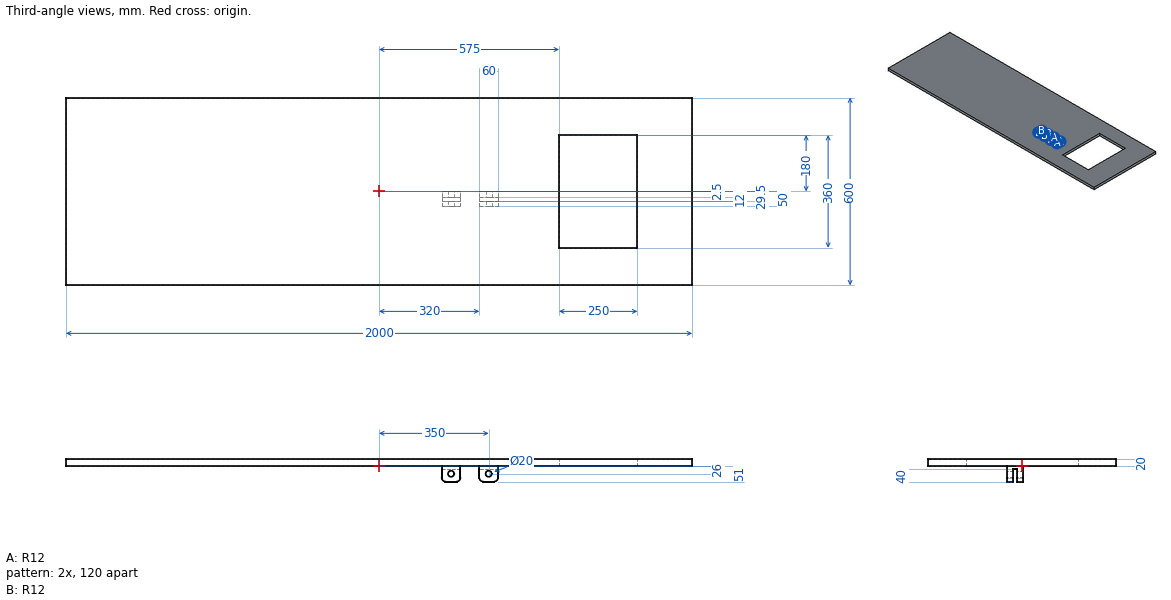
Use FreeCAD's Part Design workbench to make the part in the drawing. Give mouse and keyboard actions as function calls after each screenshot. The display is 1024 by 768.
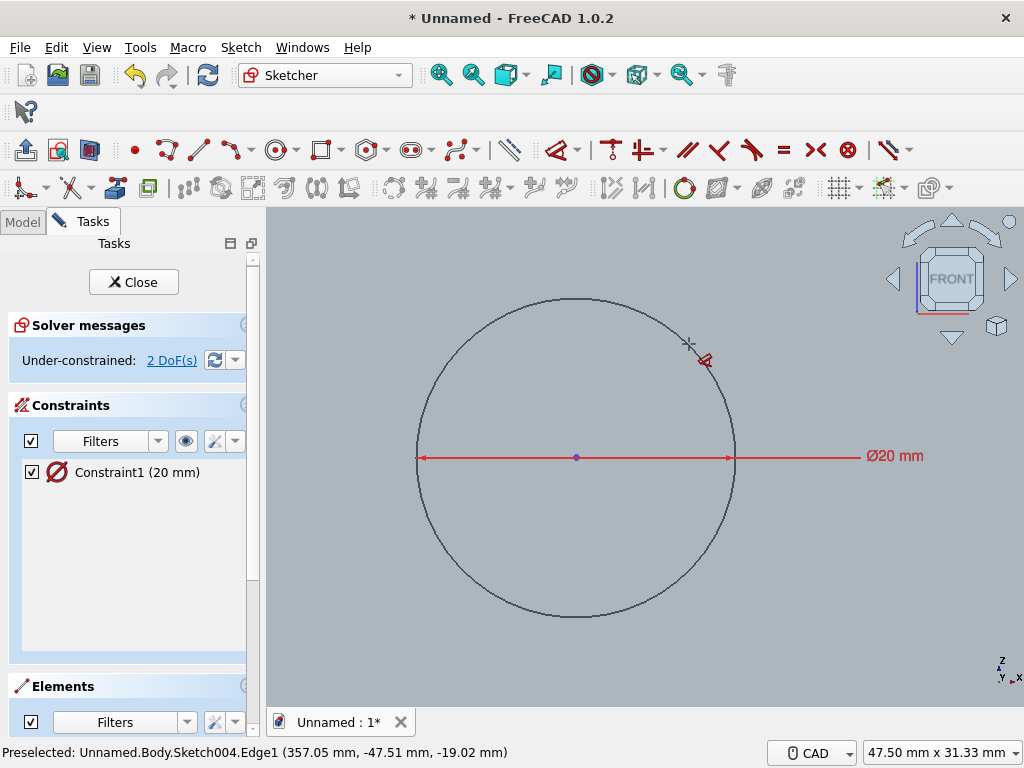
click(576, 458)
click(610, 347)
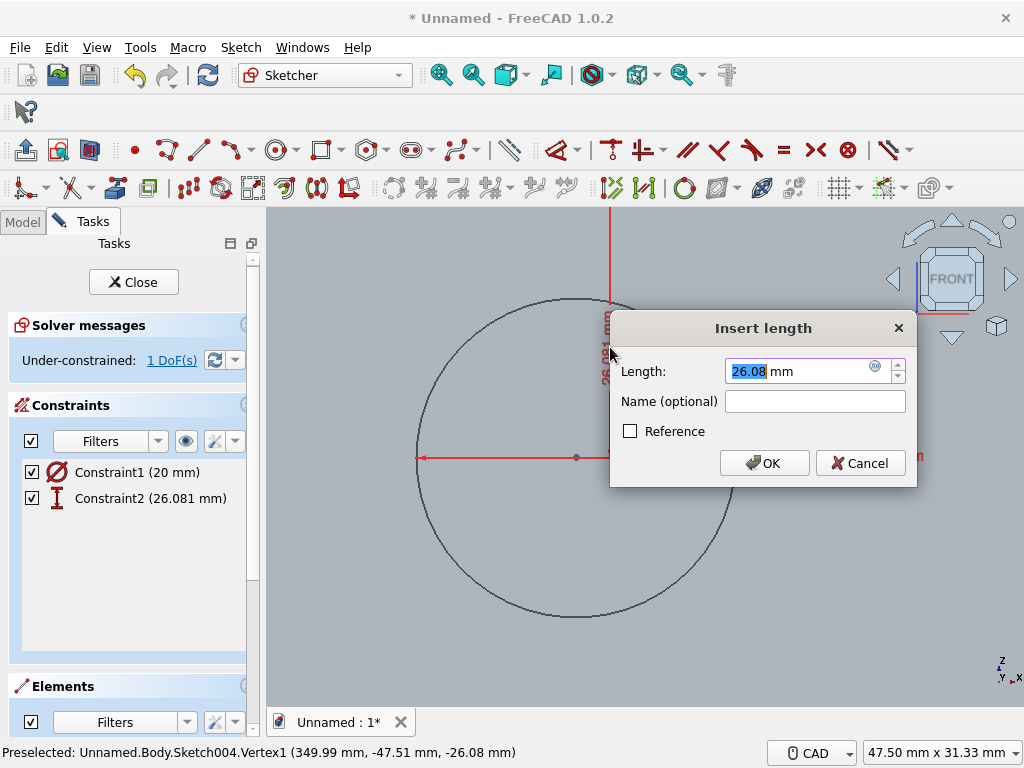
text(26)
key(Return)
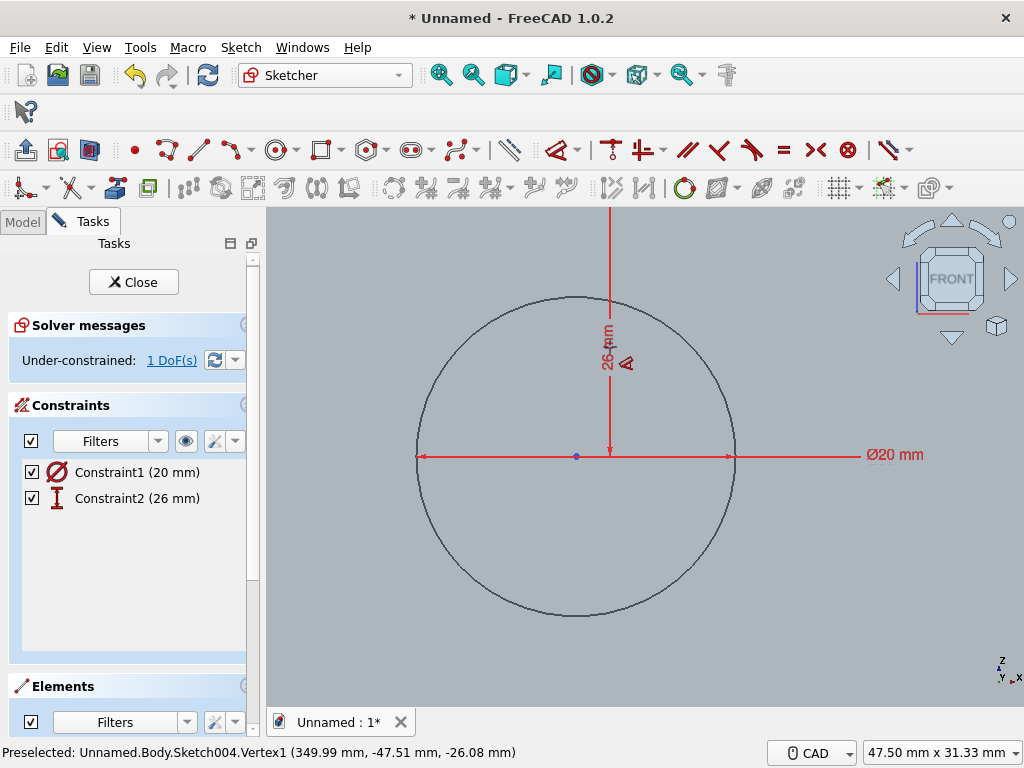
click(576, 457)
click(435, 491)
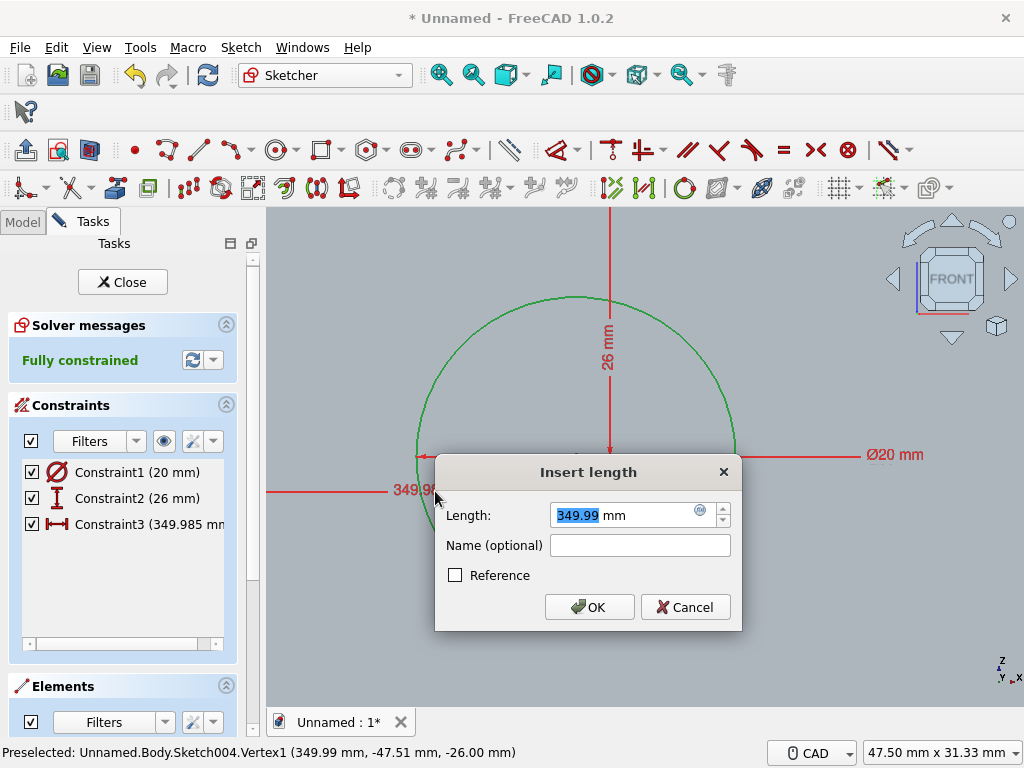
text(350)
key(Return)
key(Escape)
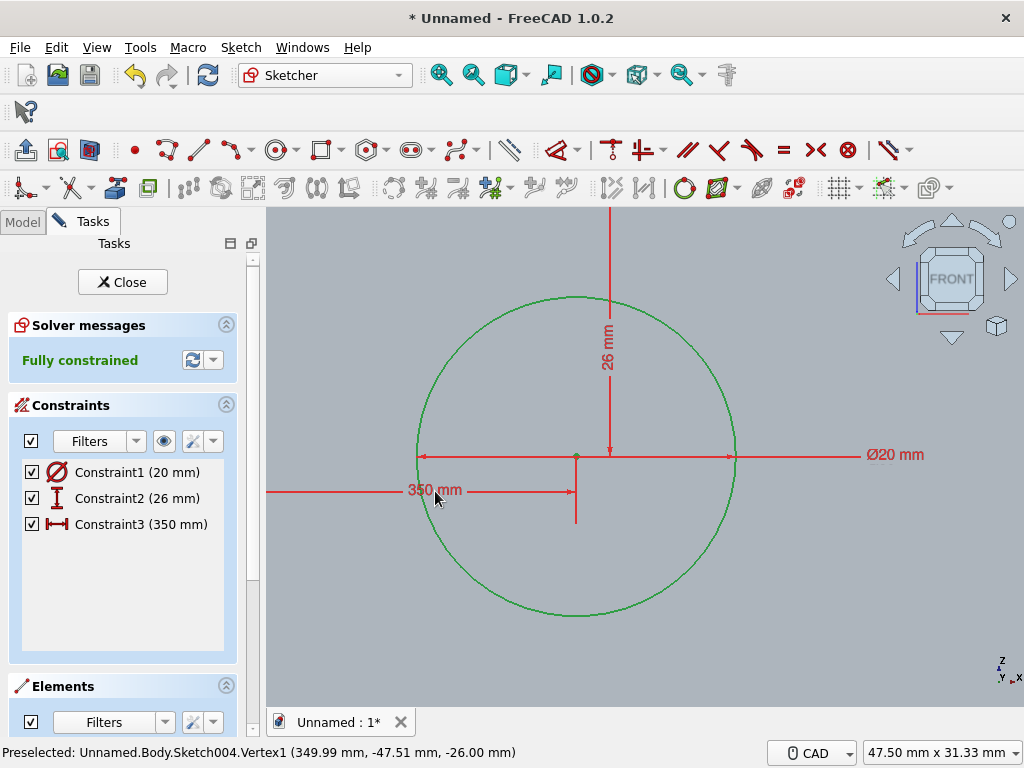
click(123, 282)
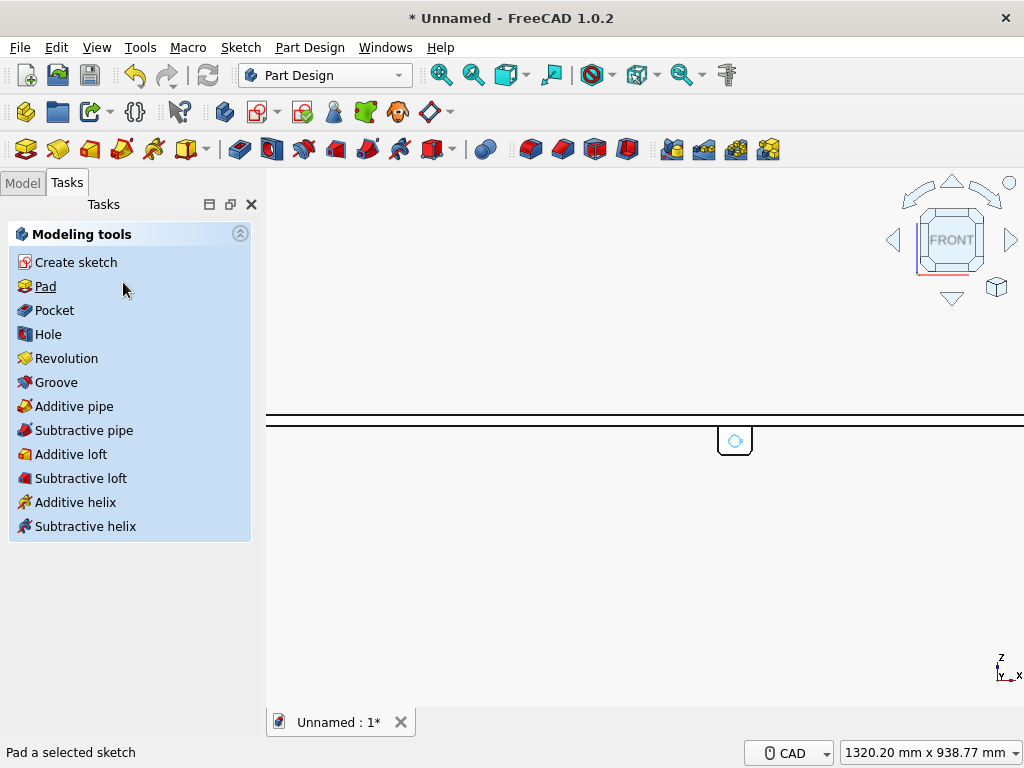
click(240, 150)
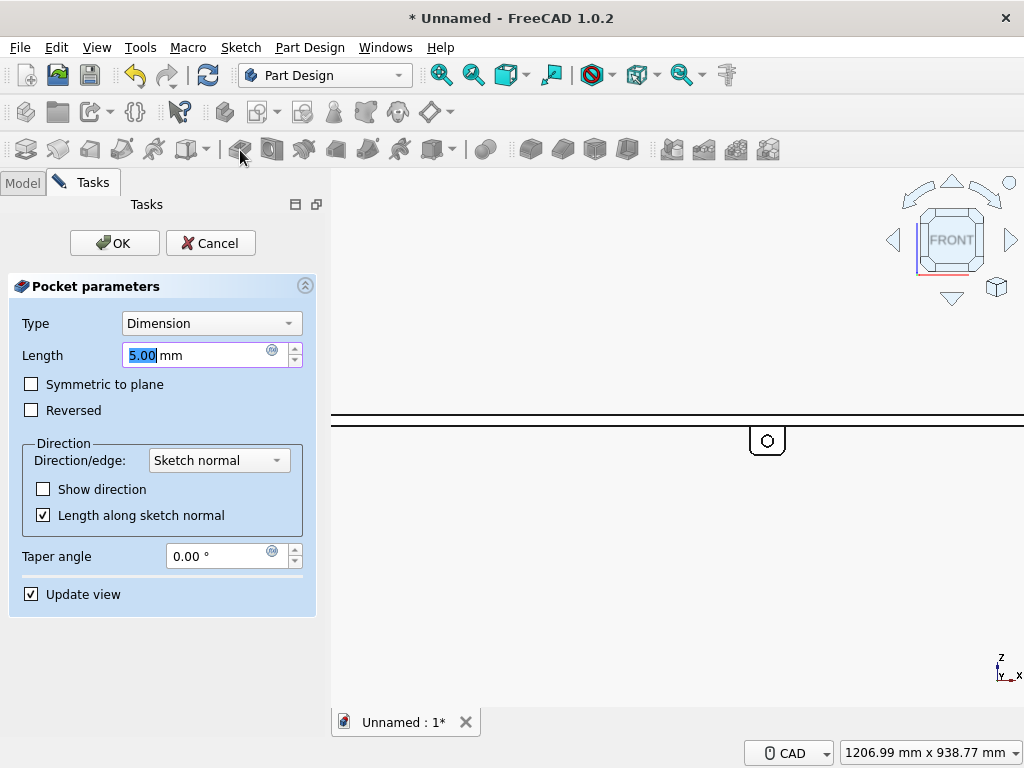
click(212, 324)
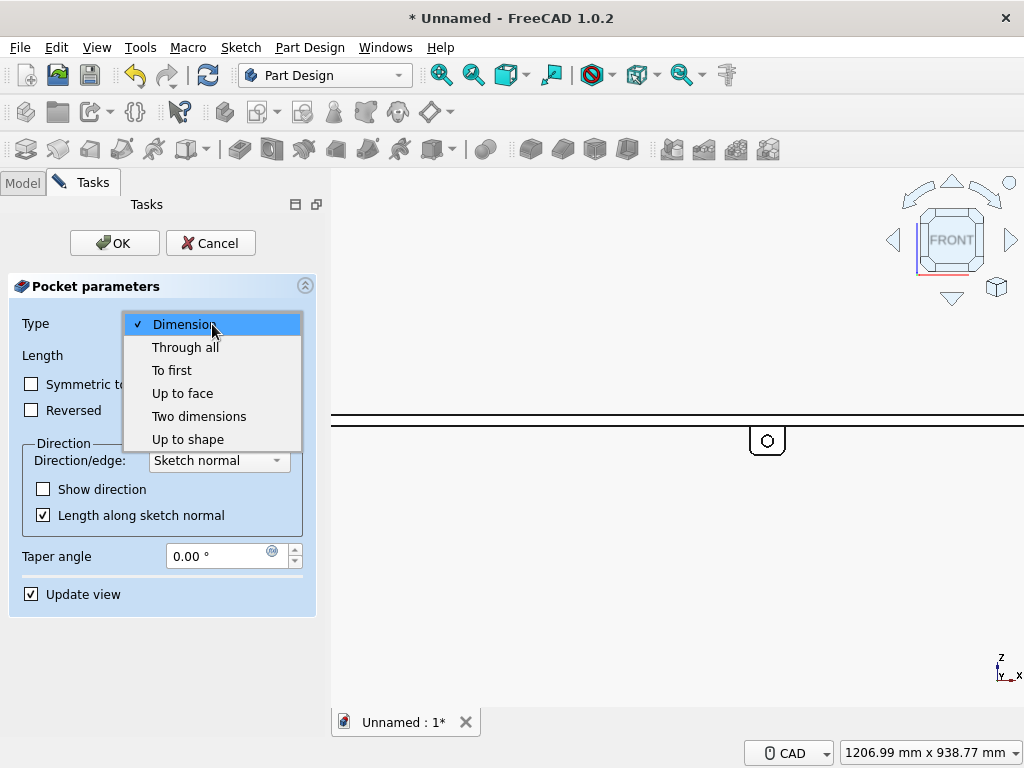
click(212, 348)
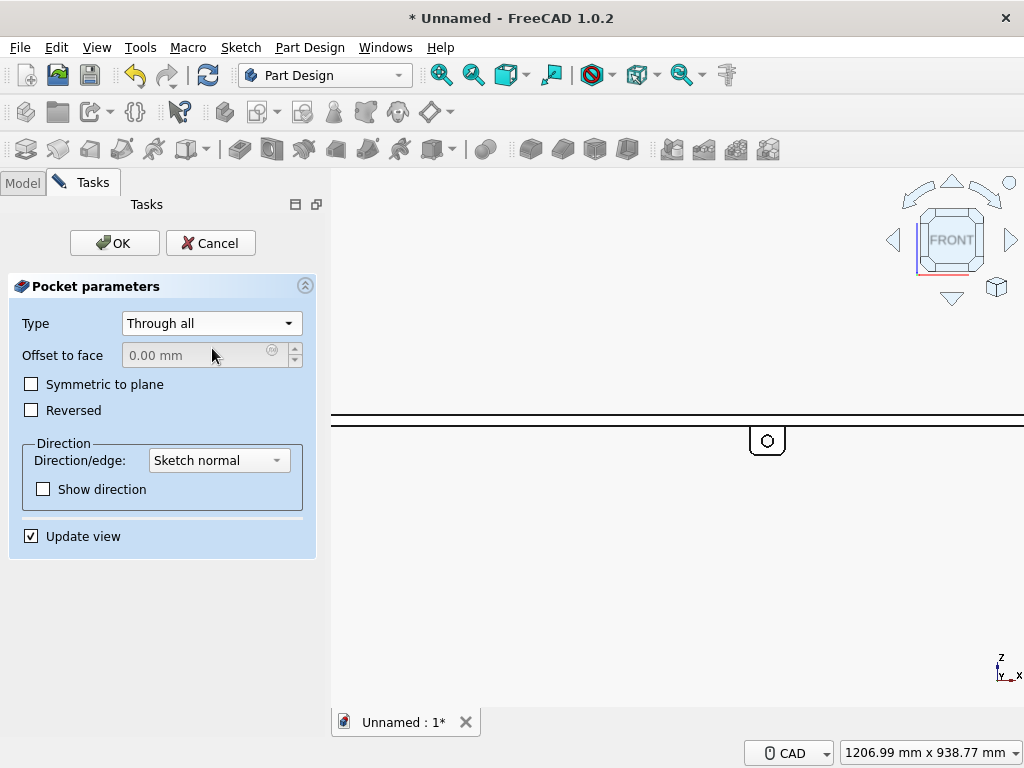
click(115, 243)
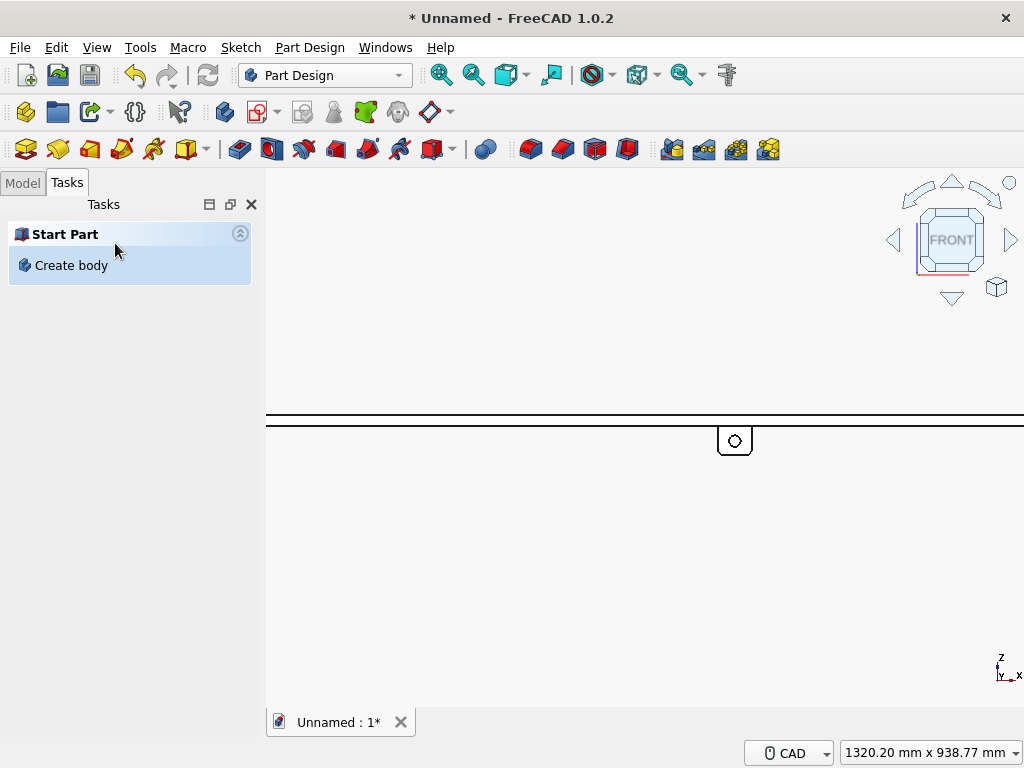
click(442, 76)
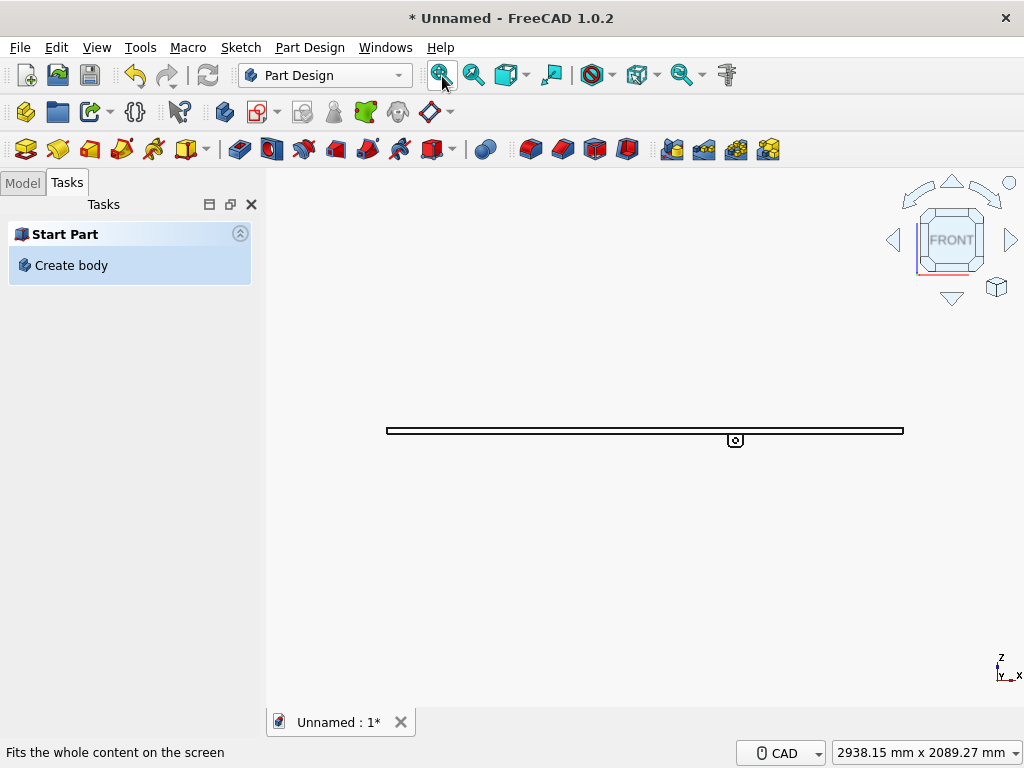
click(23, 182)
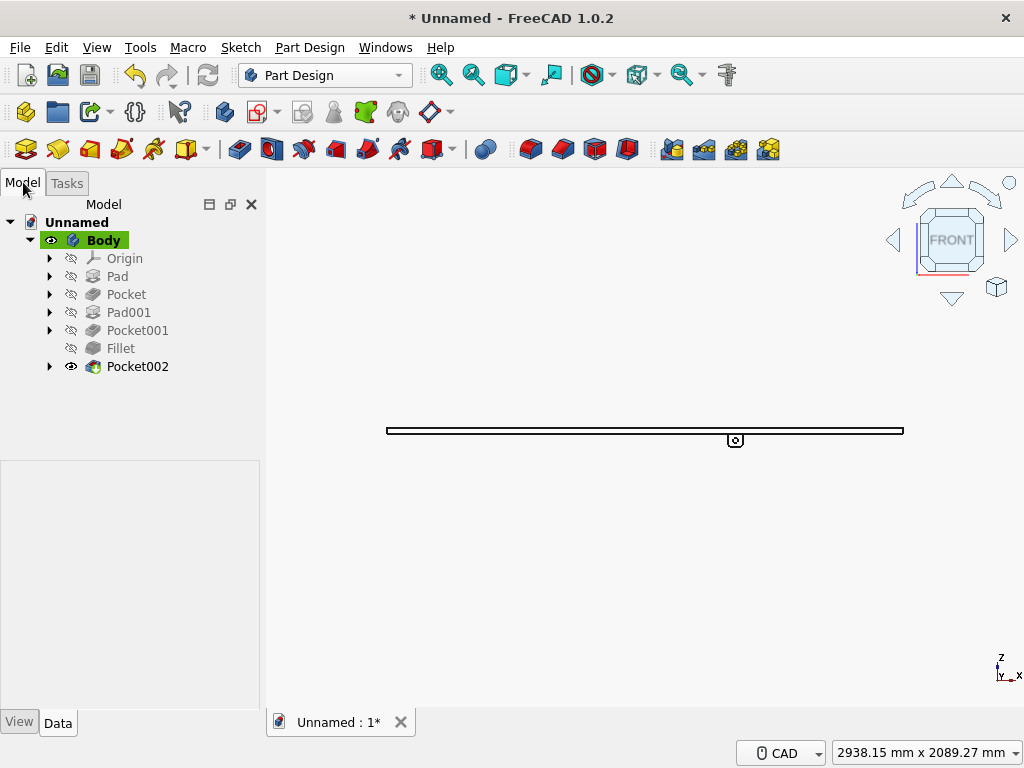
click(116, 312)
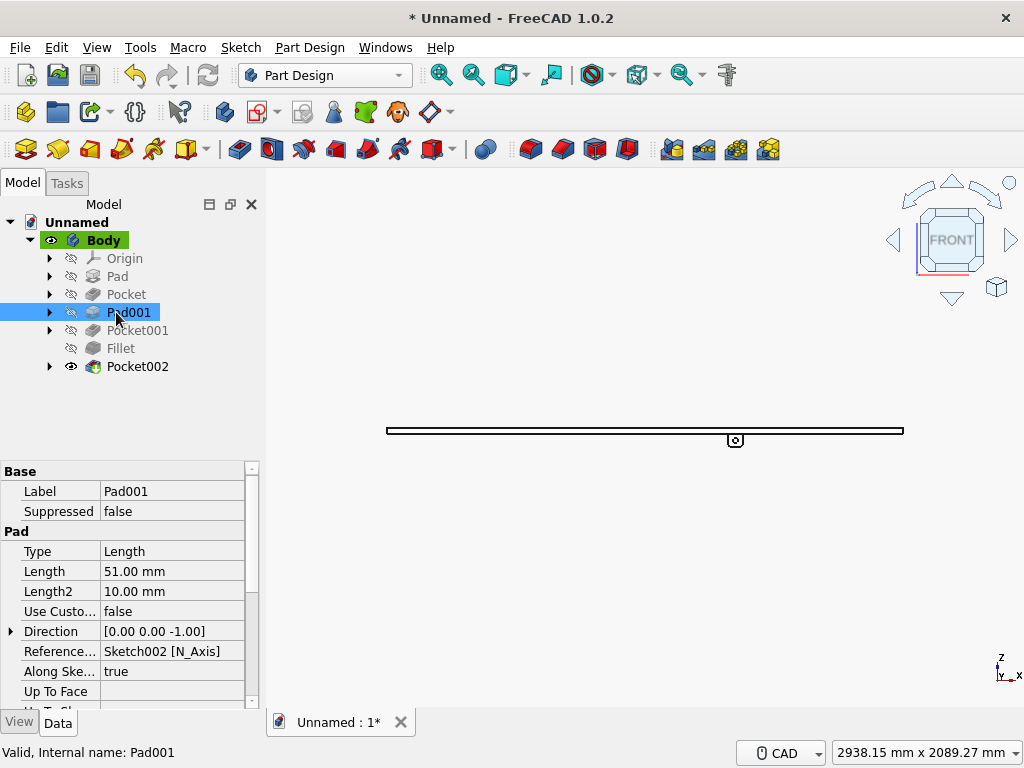
click(116, 330, ctrl)